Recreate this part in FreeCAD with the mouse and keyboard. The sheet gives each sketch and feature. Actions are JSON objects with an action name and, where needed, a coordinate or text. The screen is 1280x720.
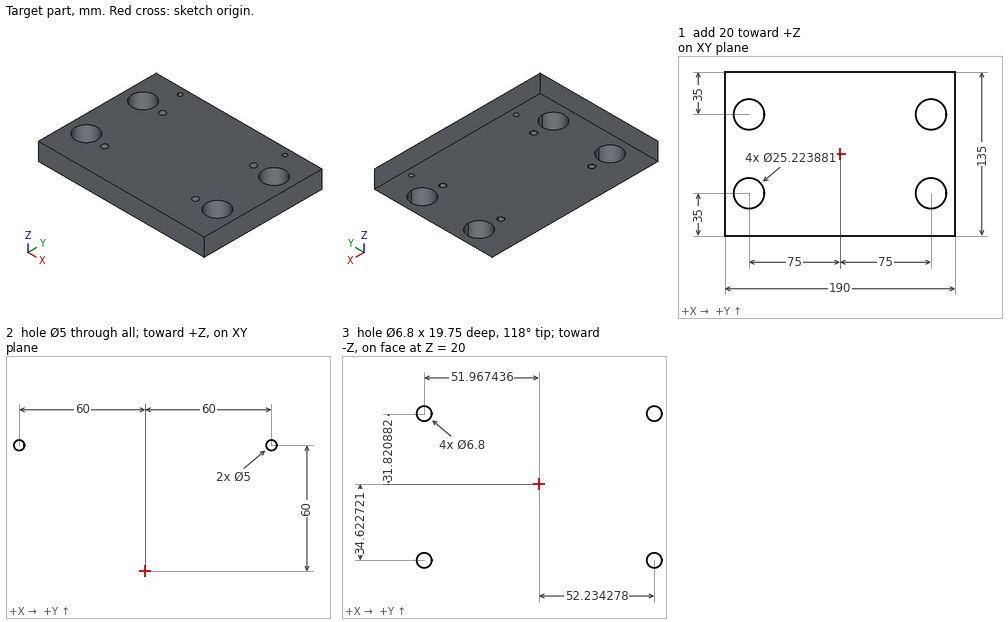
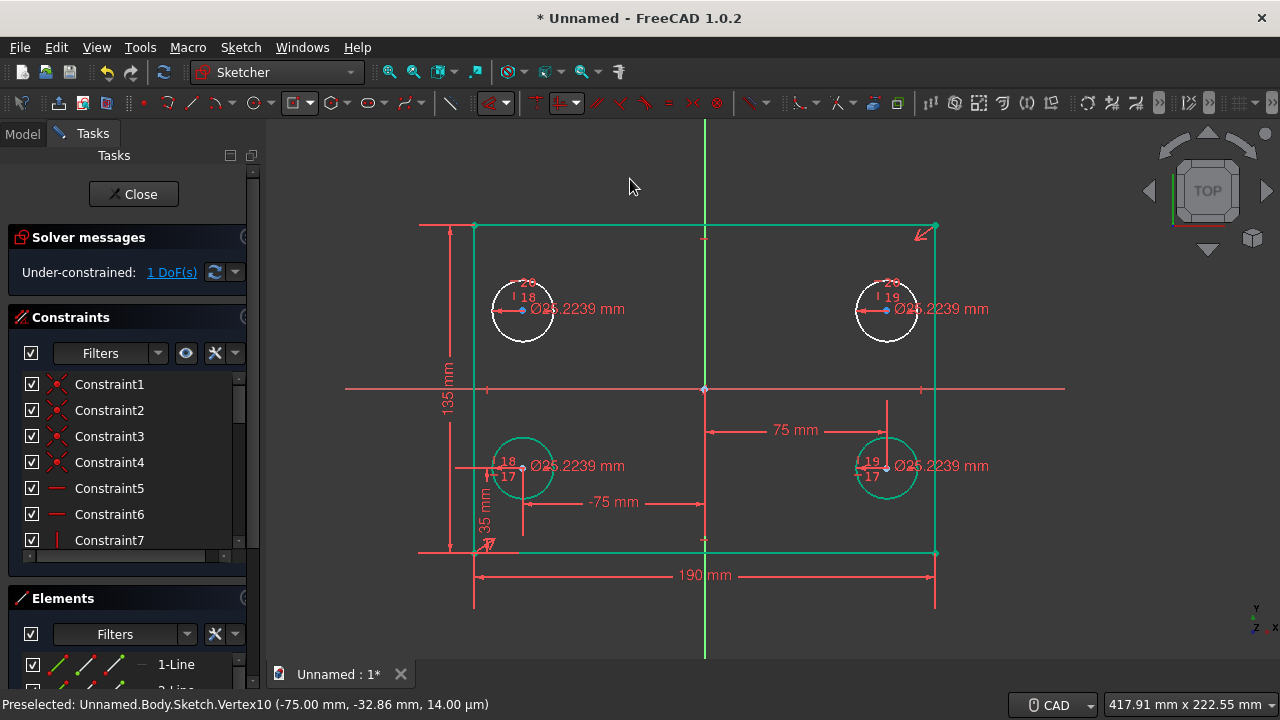
{"action": "left_click", "coordinate": [474, 225]}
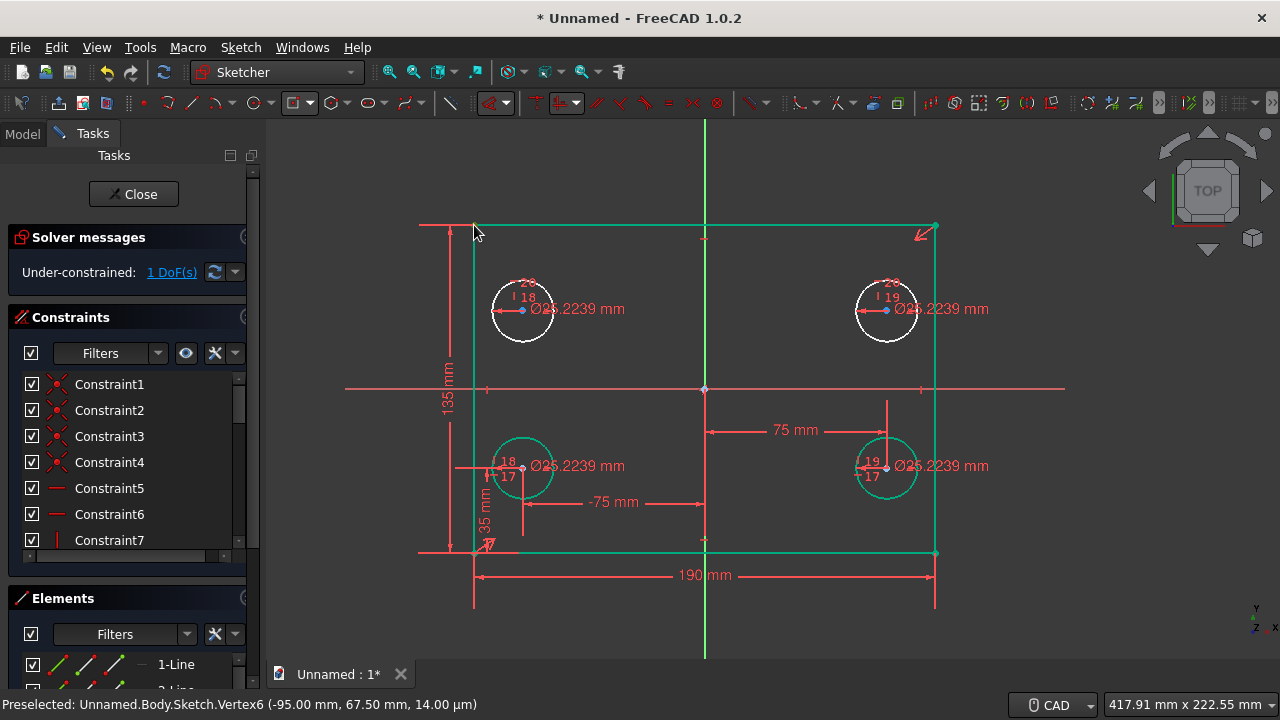
{"action": "left_click", "coordinate": [523, 311]}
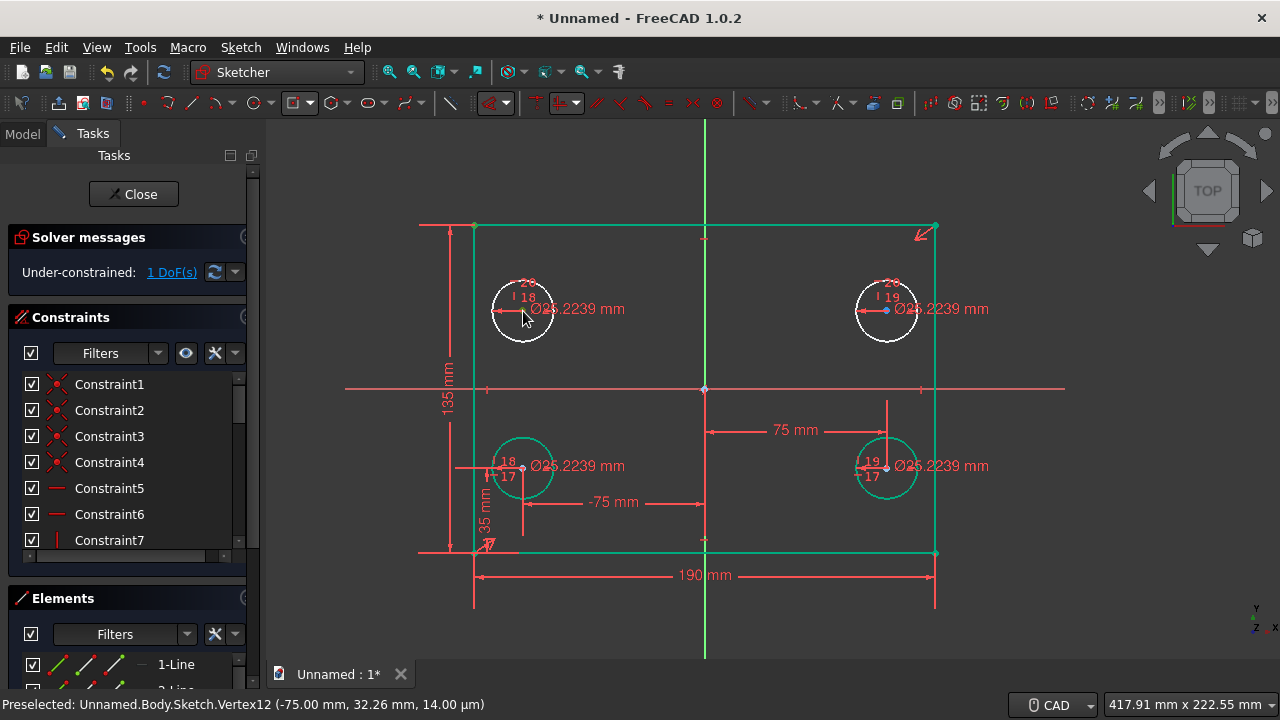
{"action": "left_click", "coordinate": [508, 104]}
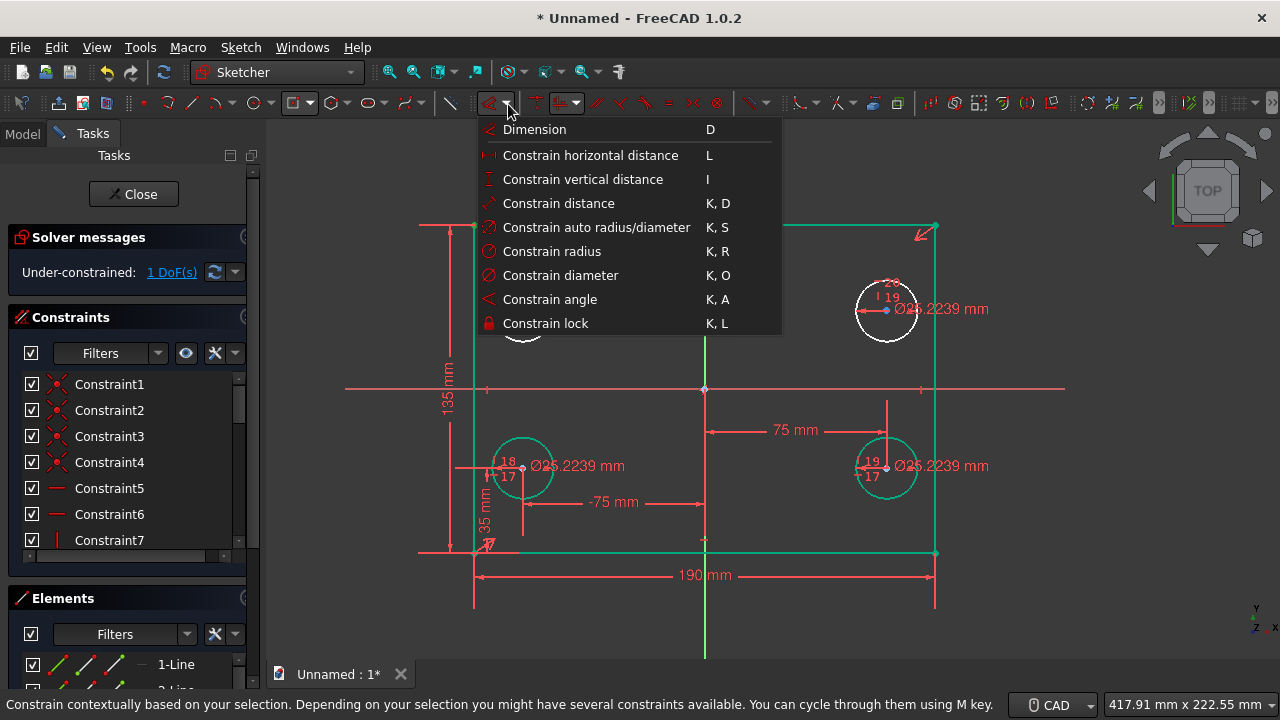
{"action": "left_click", "coordinate": [630, 179]}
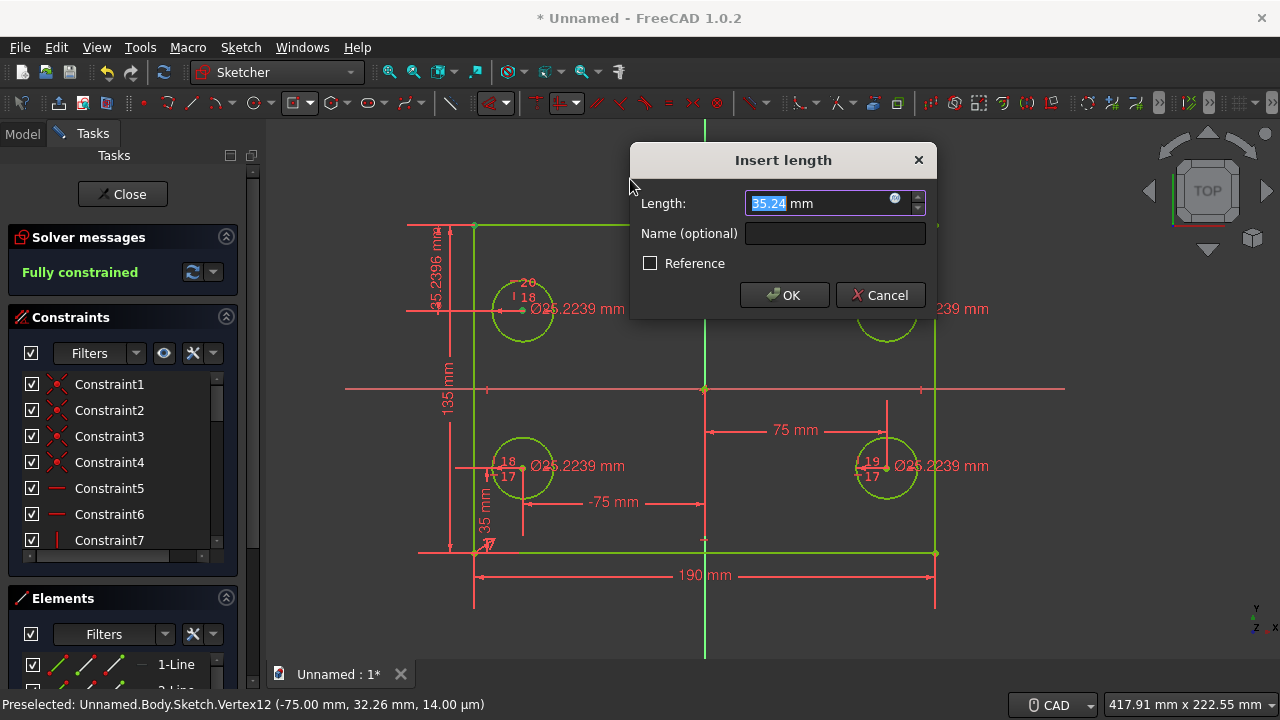
{"action": "type", "text": "35"}
{"action": "key", "text": "Return"}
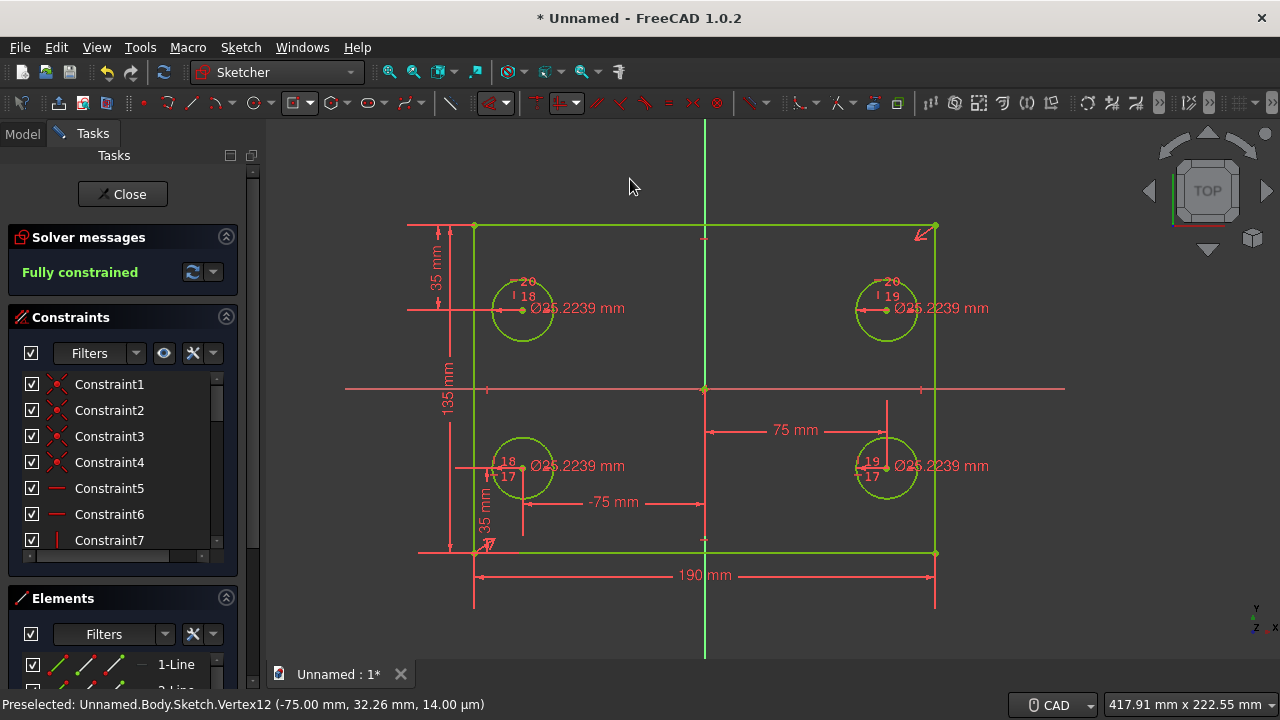
{"action": "left_click", "coordinate": [123, 194]}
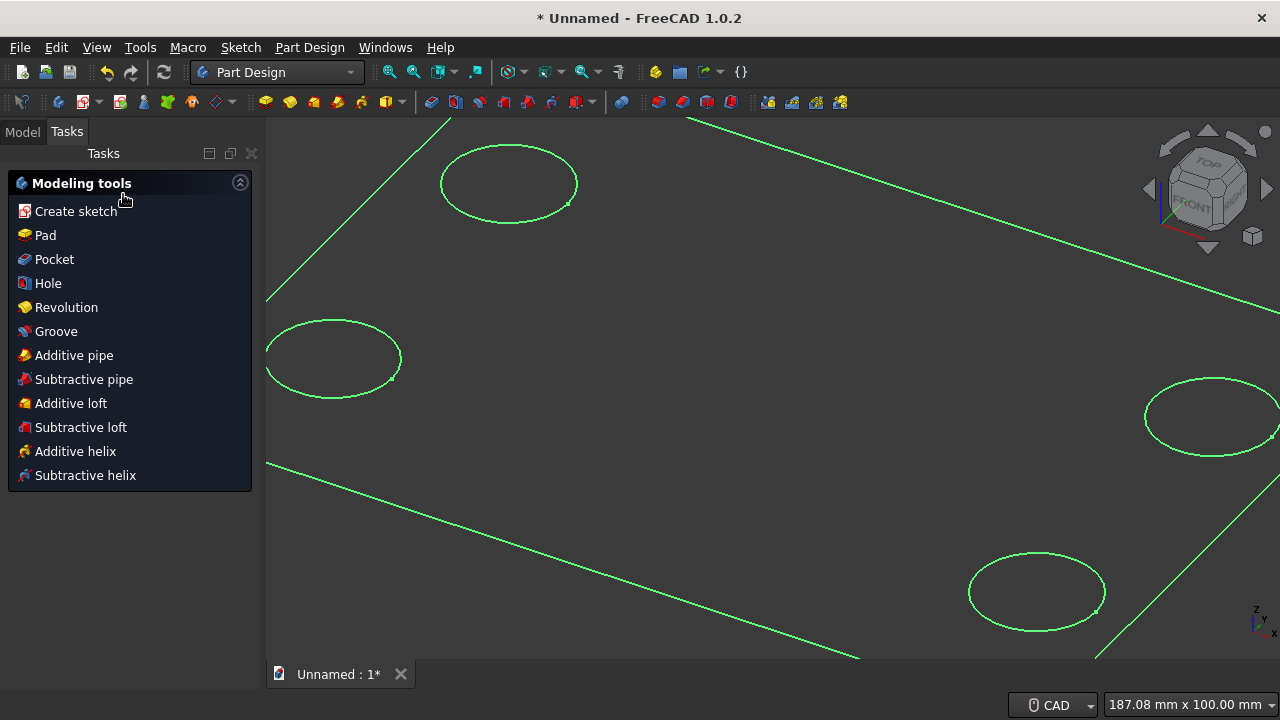
{"action": "left_click", "coordinate": [266, 102]}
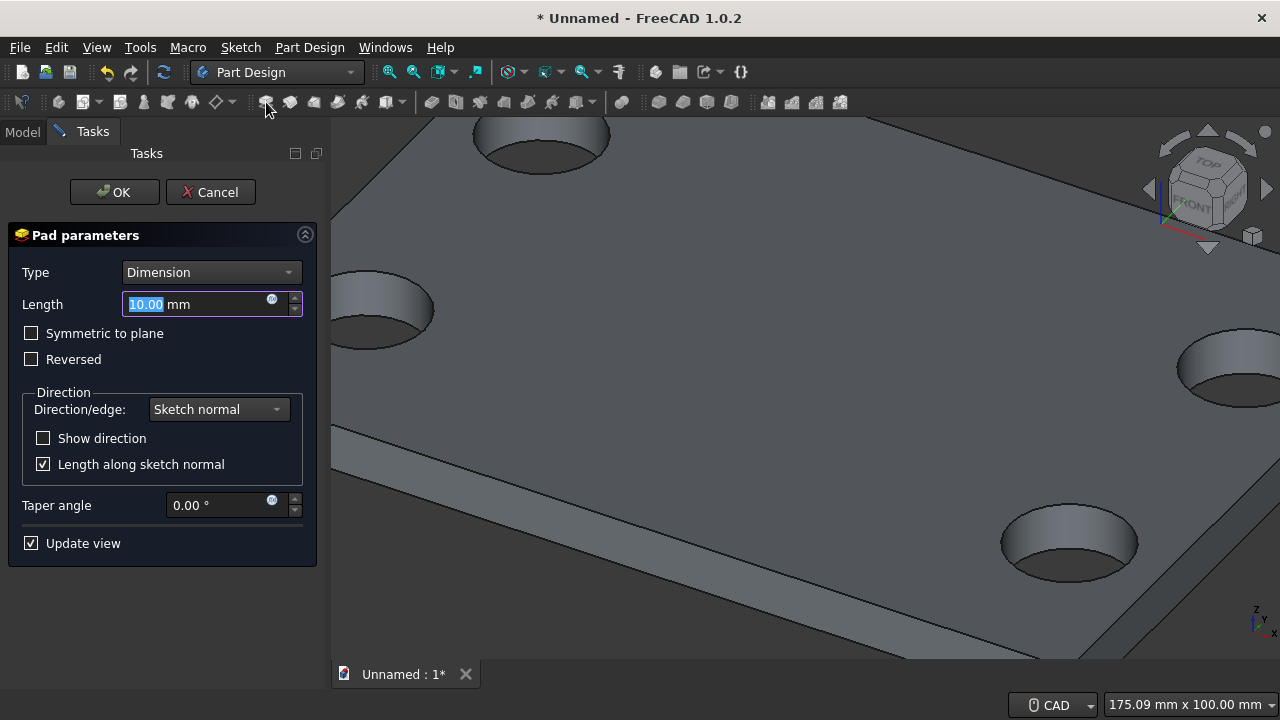
{"action": "type", "text": "20"}
{"action": "key", "text": "Tab"}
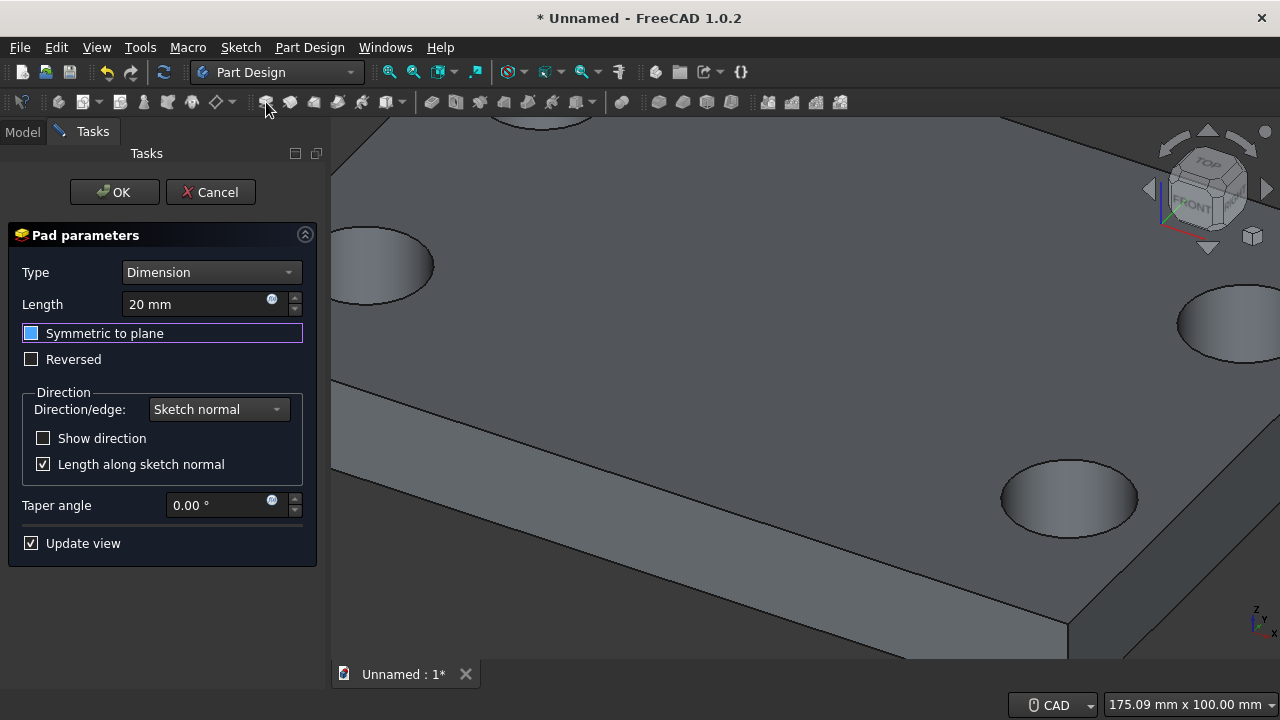
{"action": "left_click", "coordinate": [115, 192]}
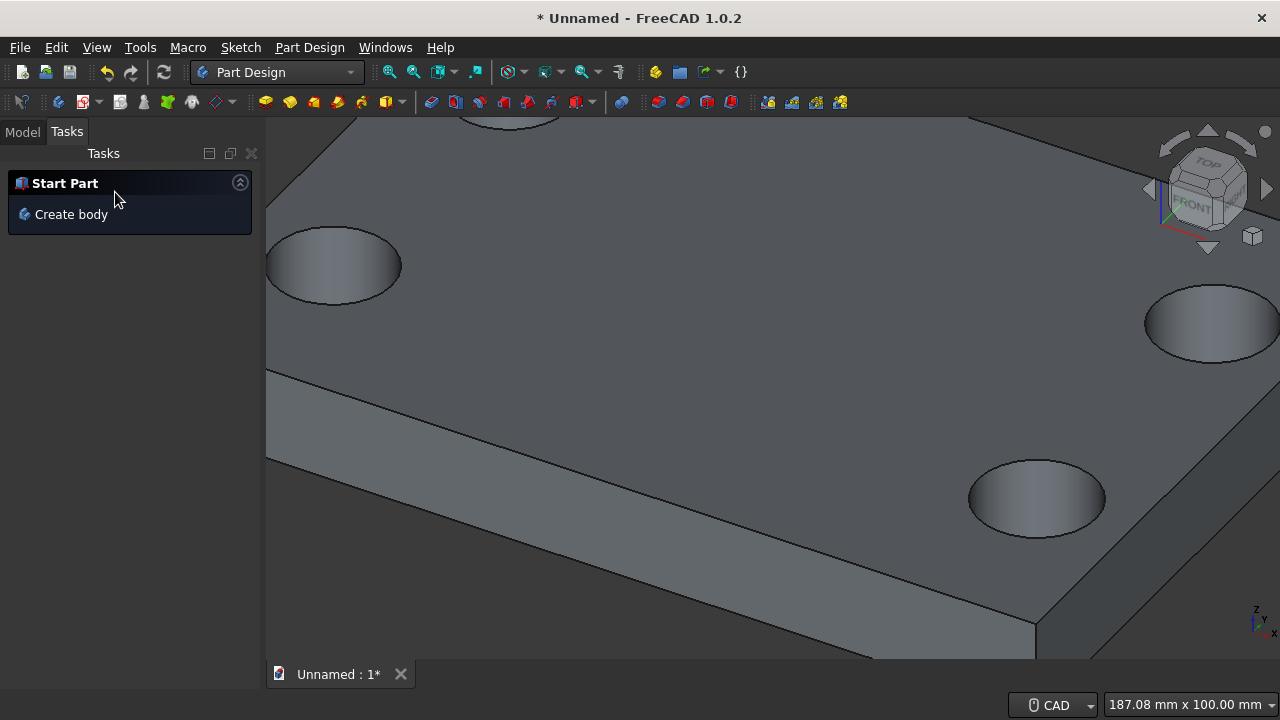
{"action": "left_click", "coordinate": [390, 72]}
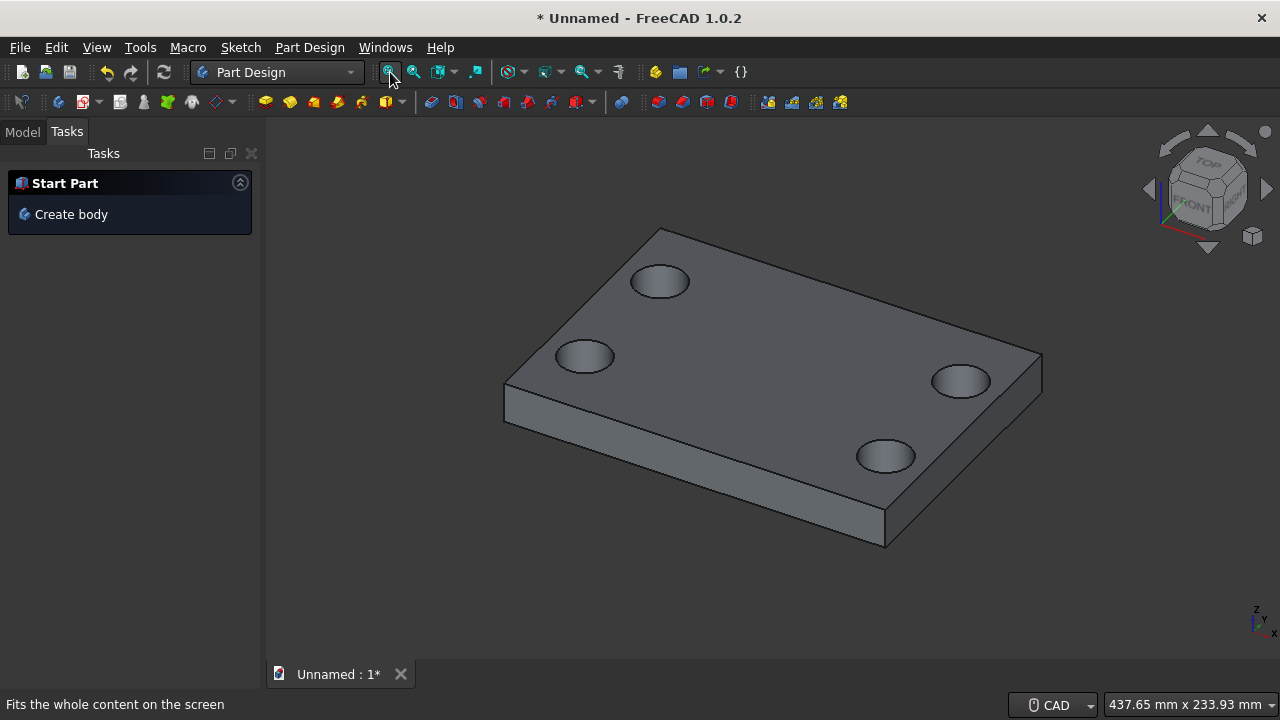
{"action": "left_click", "coordinate": [84, 102]}